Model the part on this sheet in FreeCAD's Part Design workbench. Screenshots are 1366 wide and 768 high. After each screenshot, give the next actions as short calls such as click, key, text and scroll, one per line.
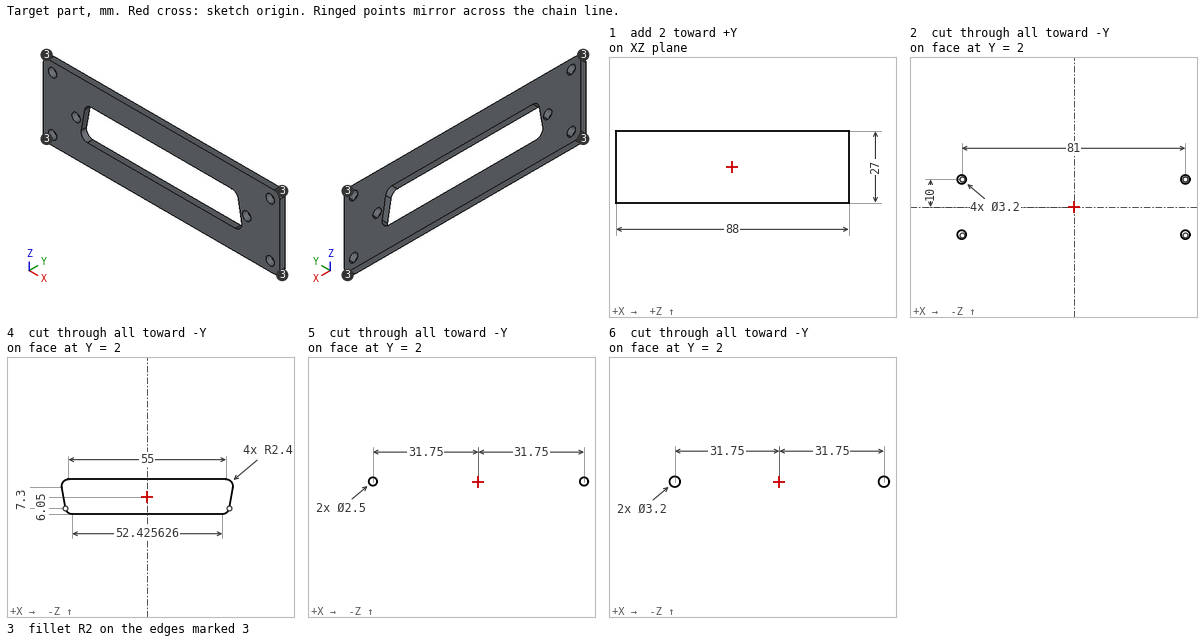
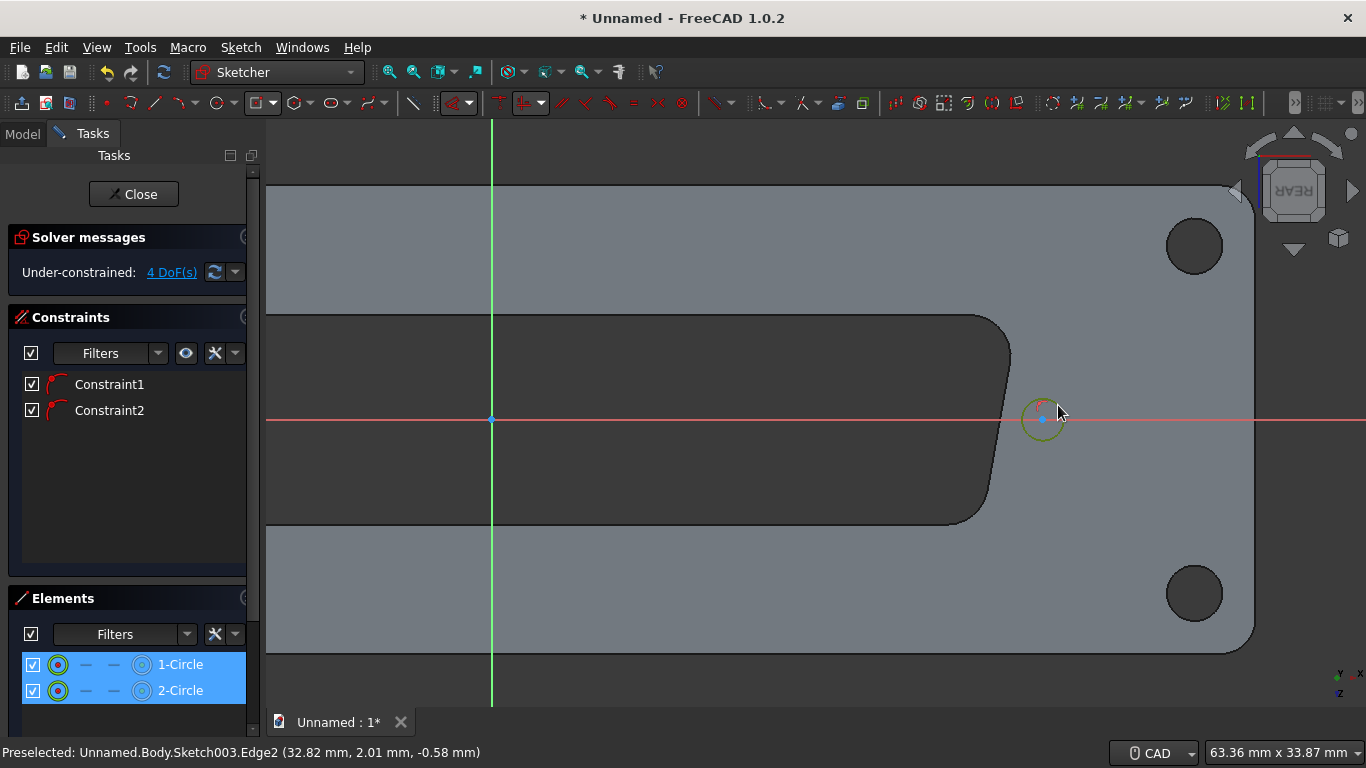
key(e)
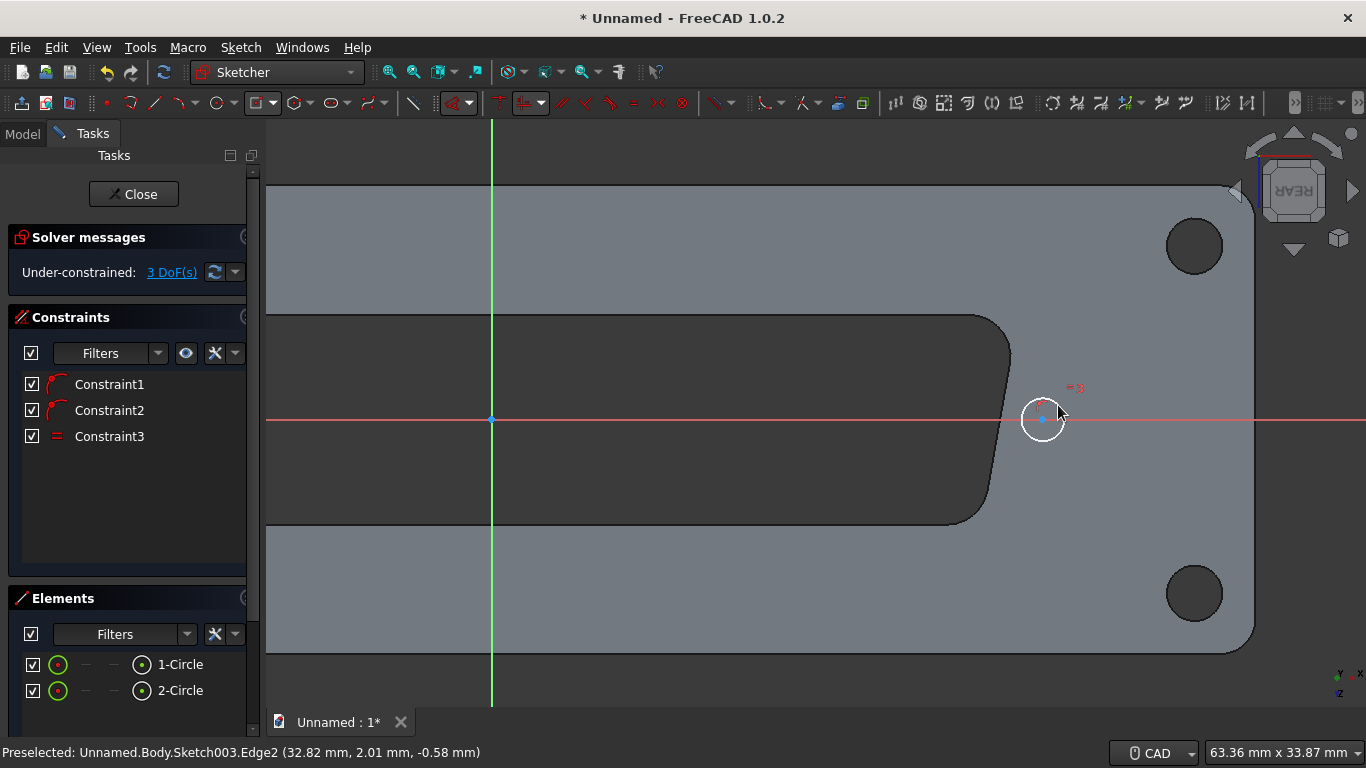
scroll(1059, 405, down, 3)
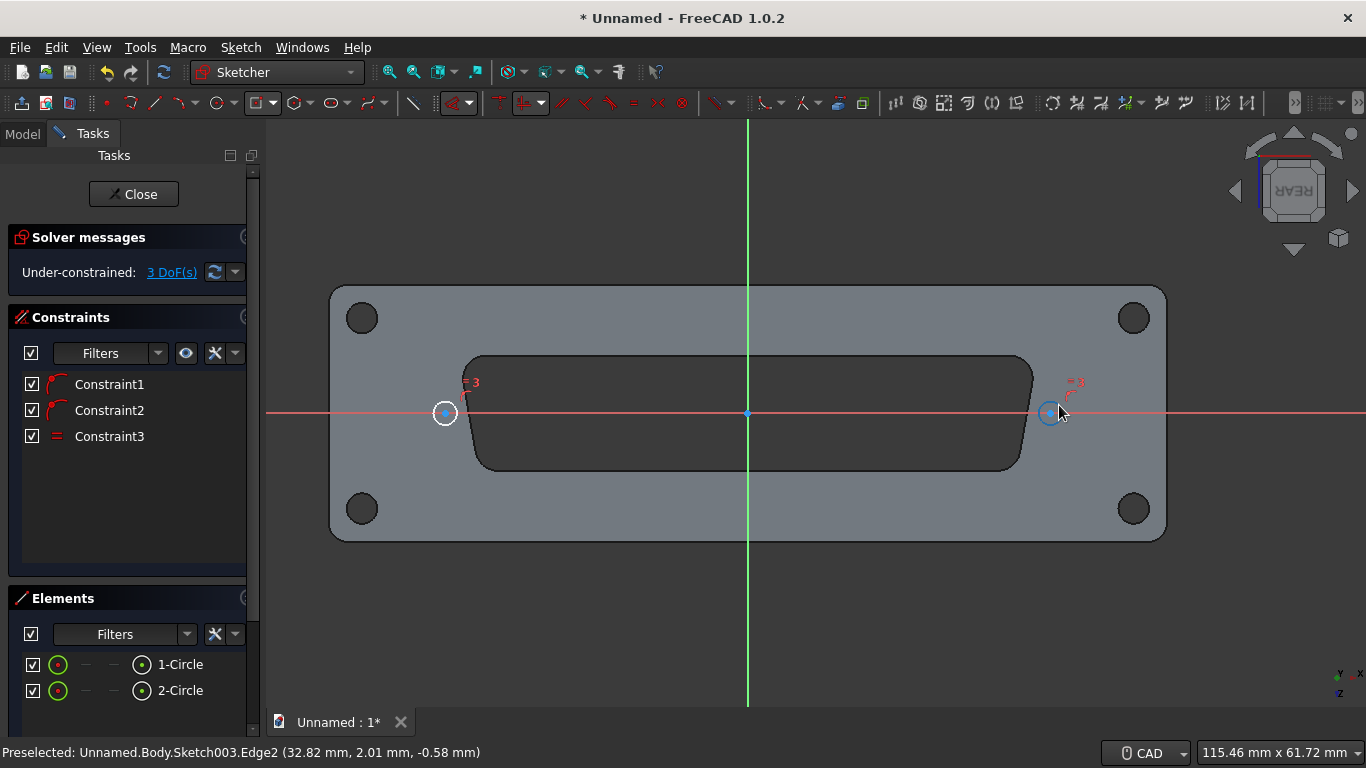
scroll(453, 405, up, 3)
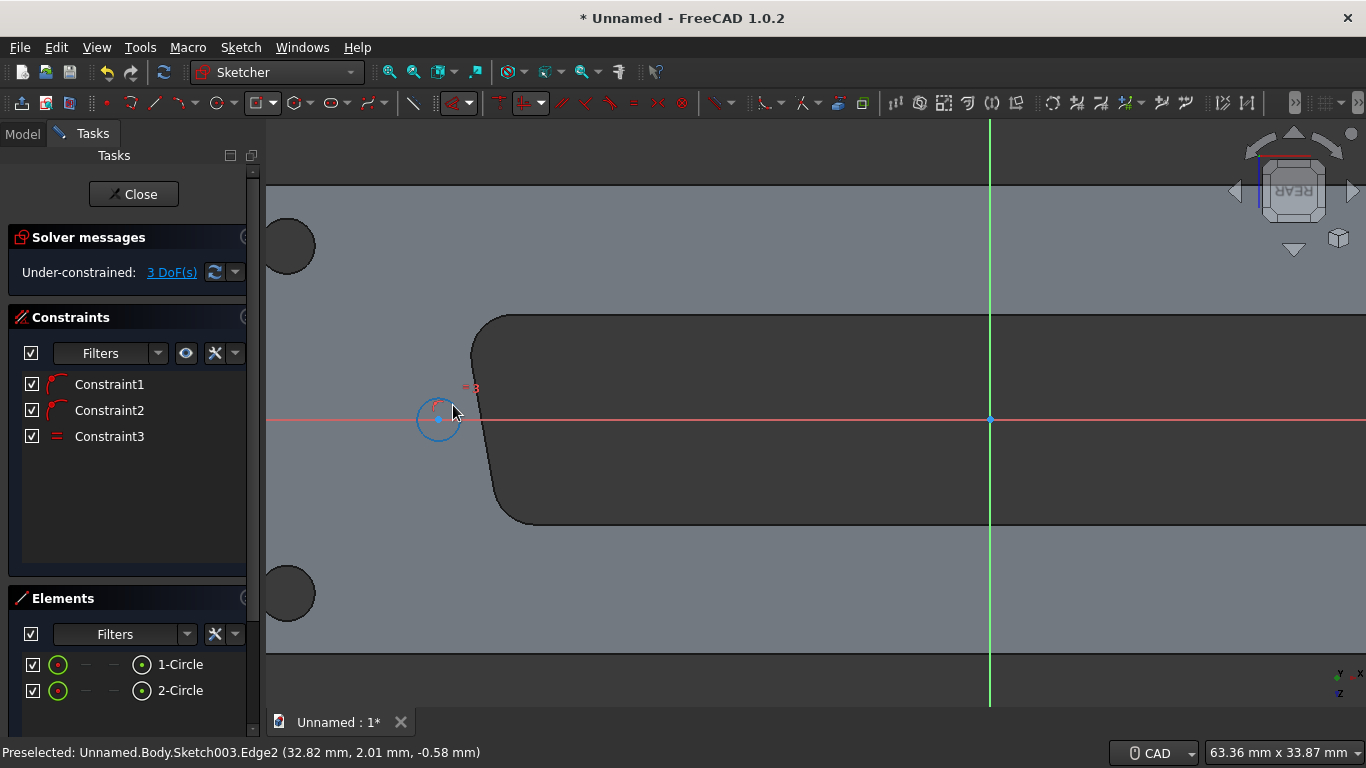
click(454, 405)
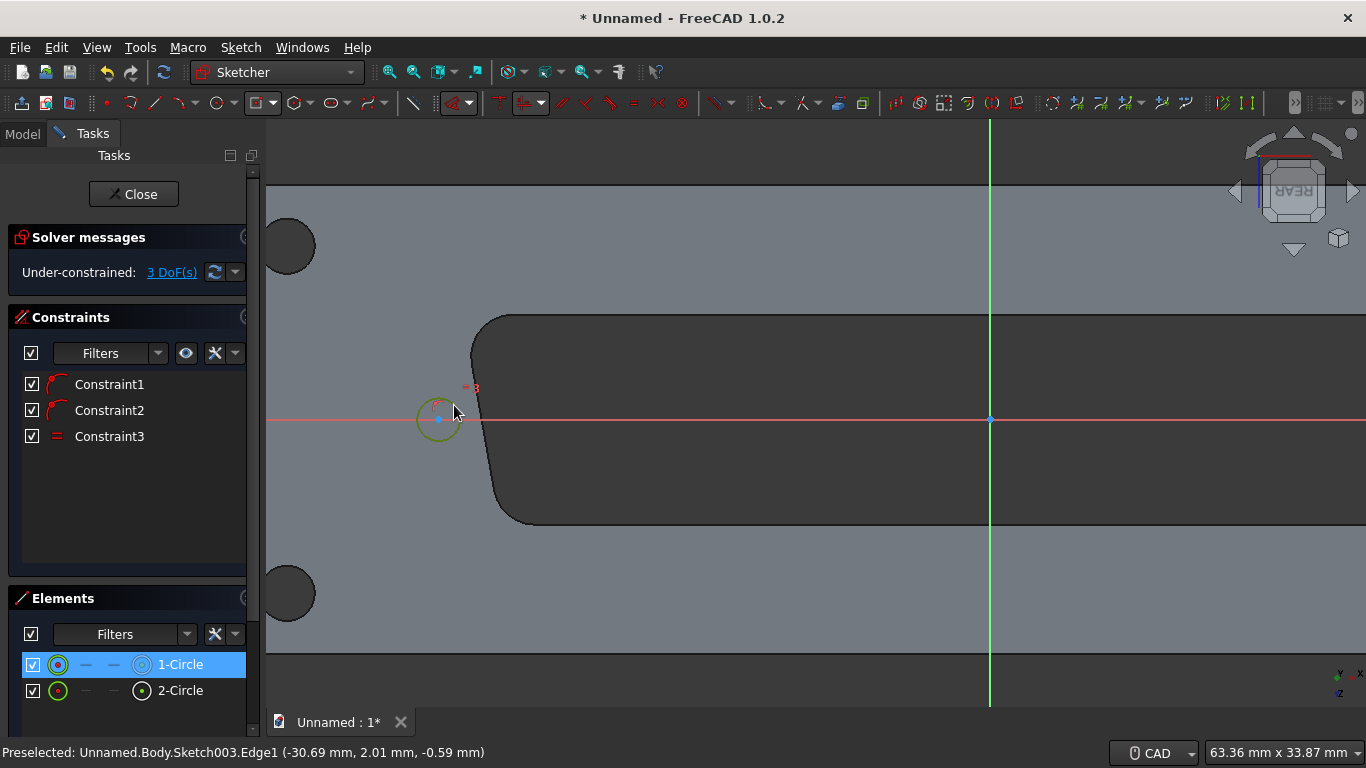
key(k)
key(o)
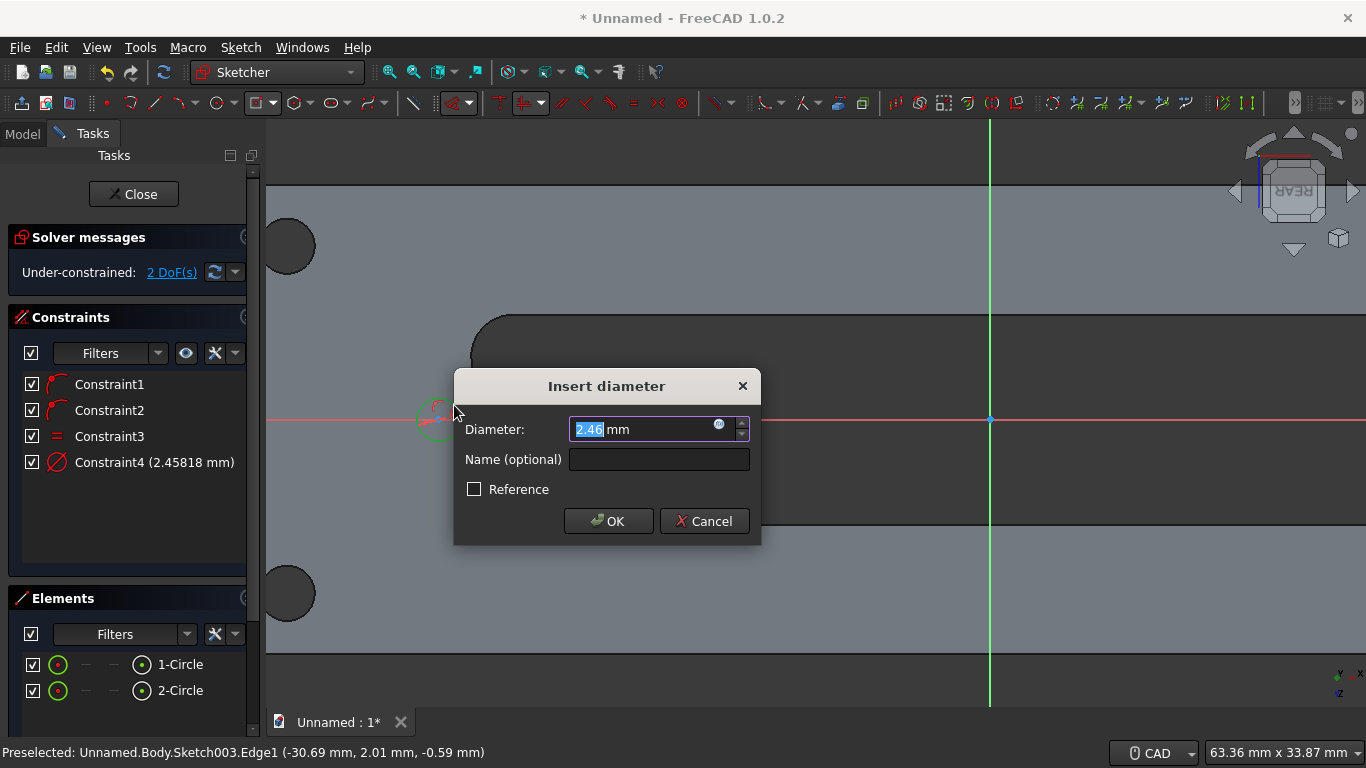
text(2.5)
key(Return)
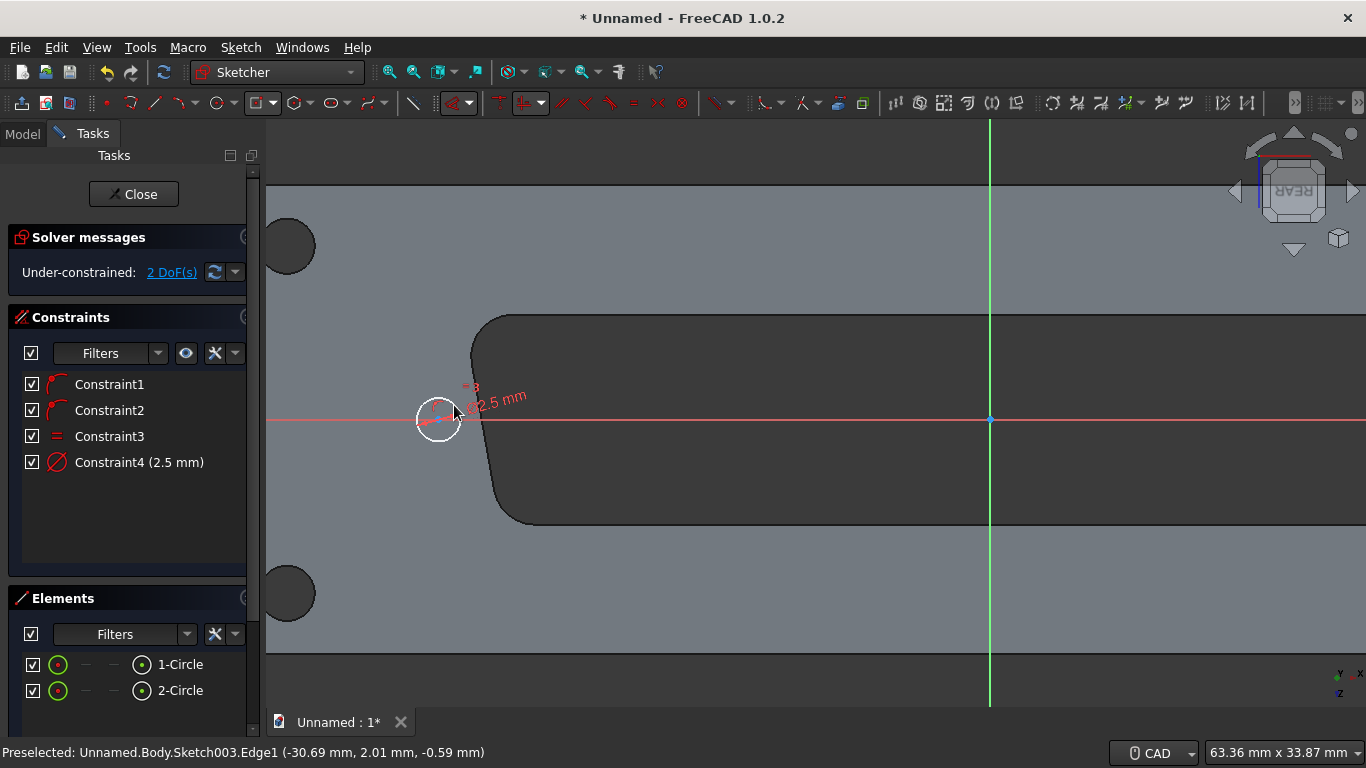
click(439, 420)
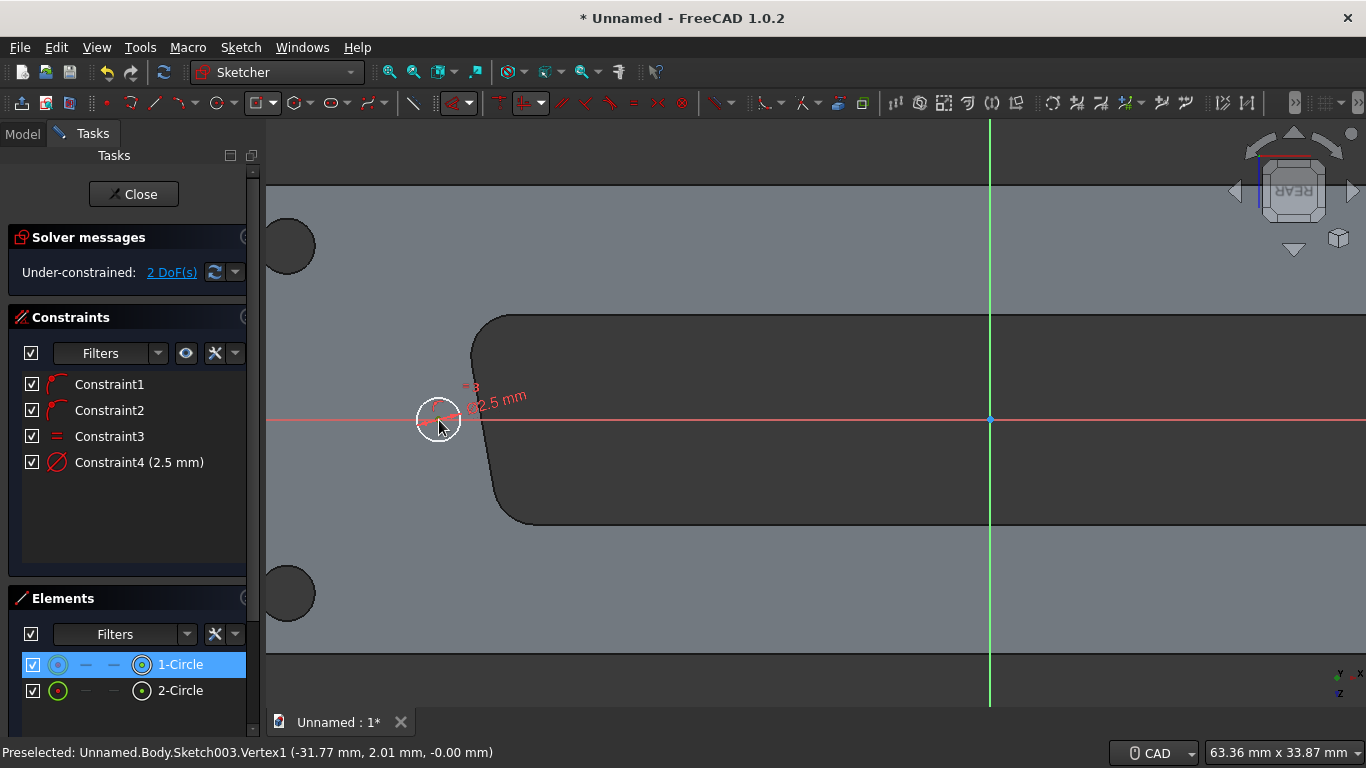
key(l)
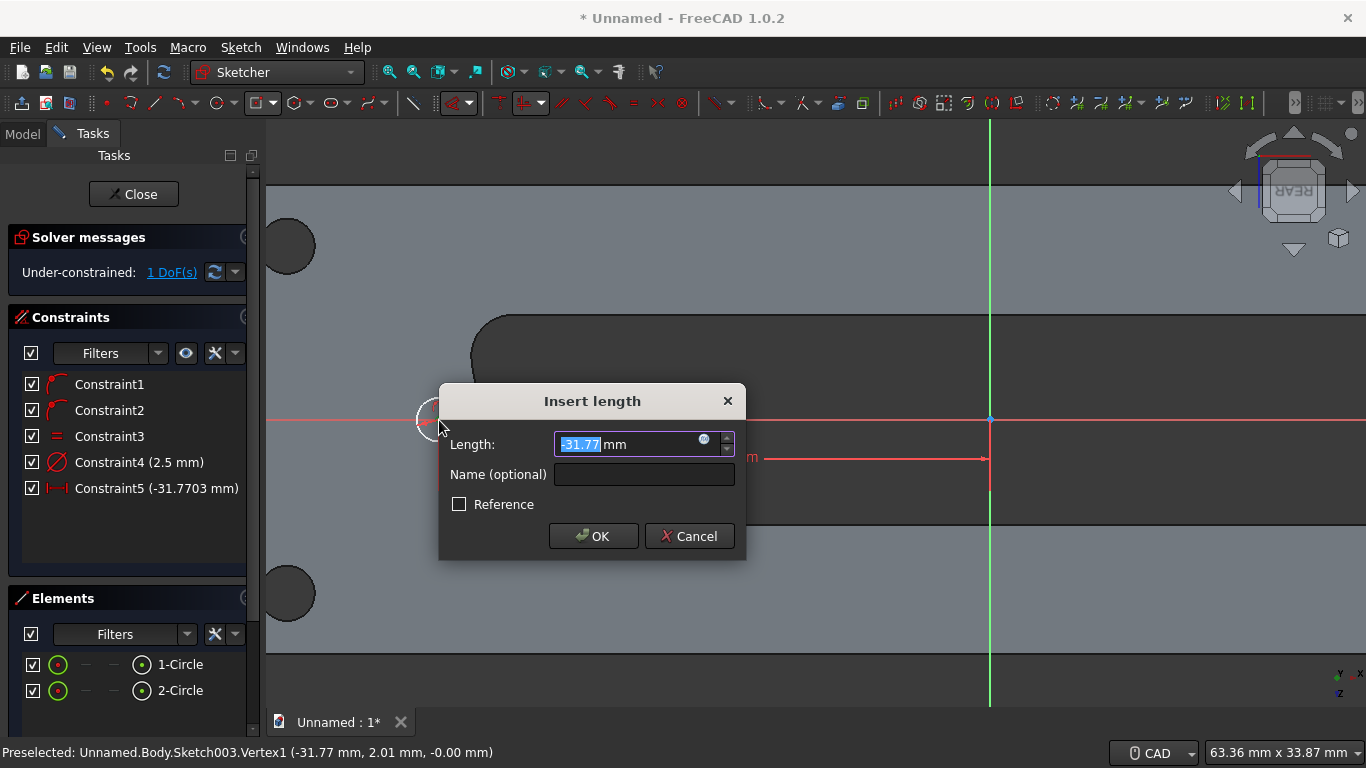
text(-31.75)
key(Return)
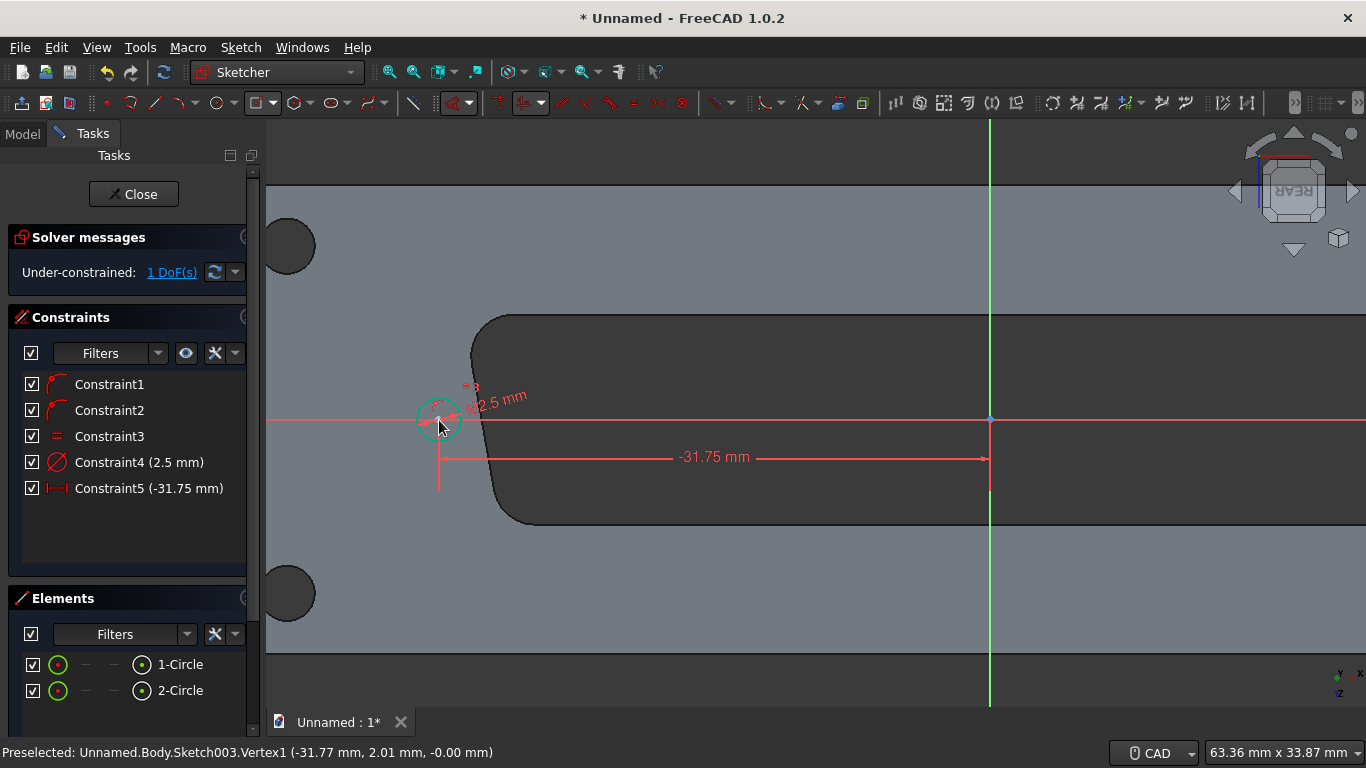
scroll(452, 405, down, 3)